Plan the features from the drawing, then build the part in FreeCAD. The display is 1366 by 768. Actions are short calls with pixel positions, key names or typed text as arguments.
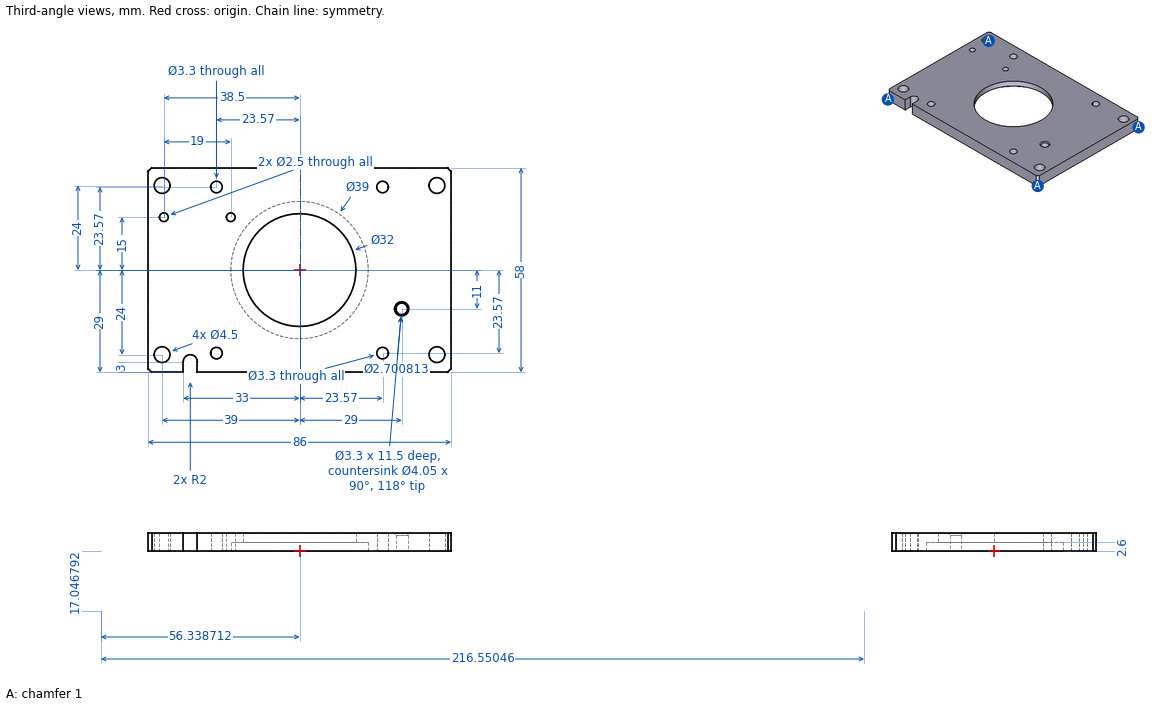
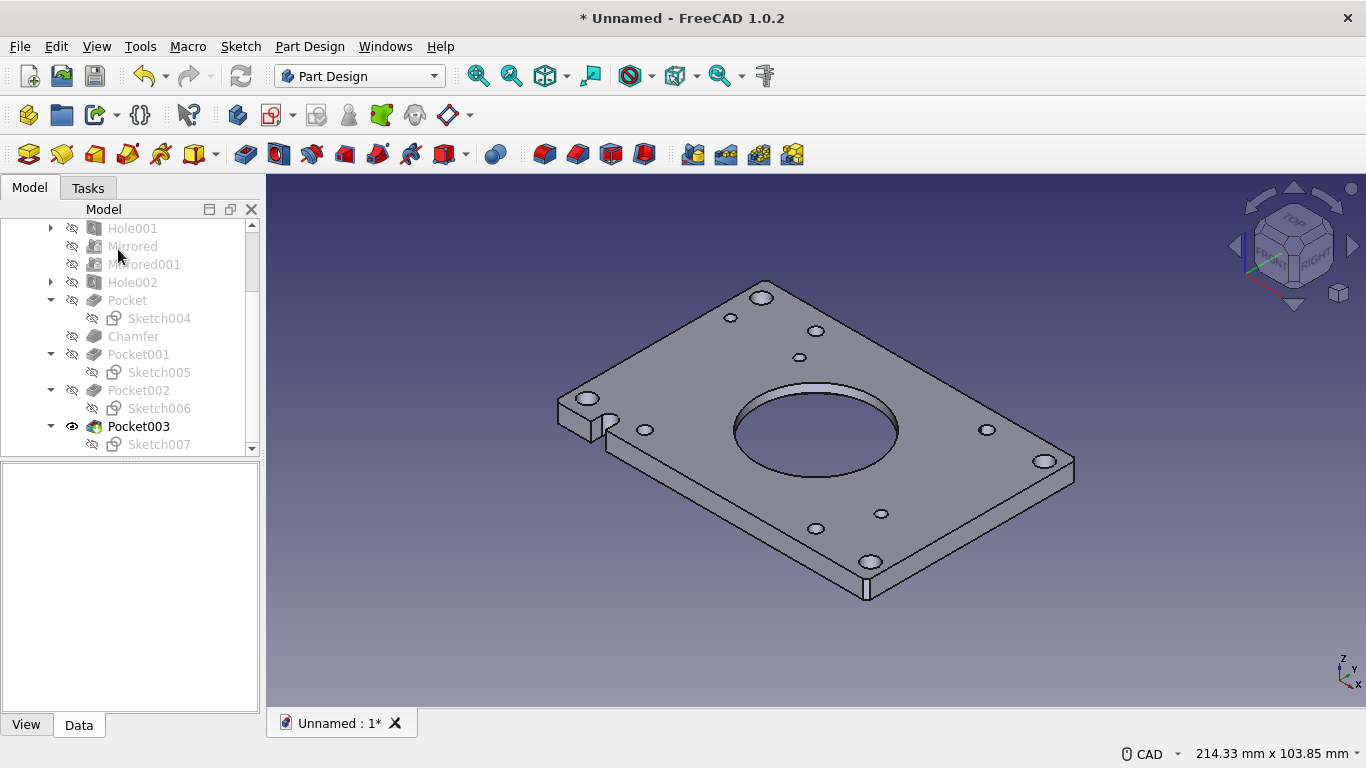
click(697, 395)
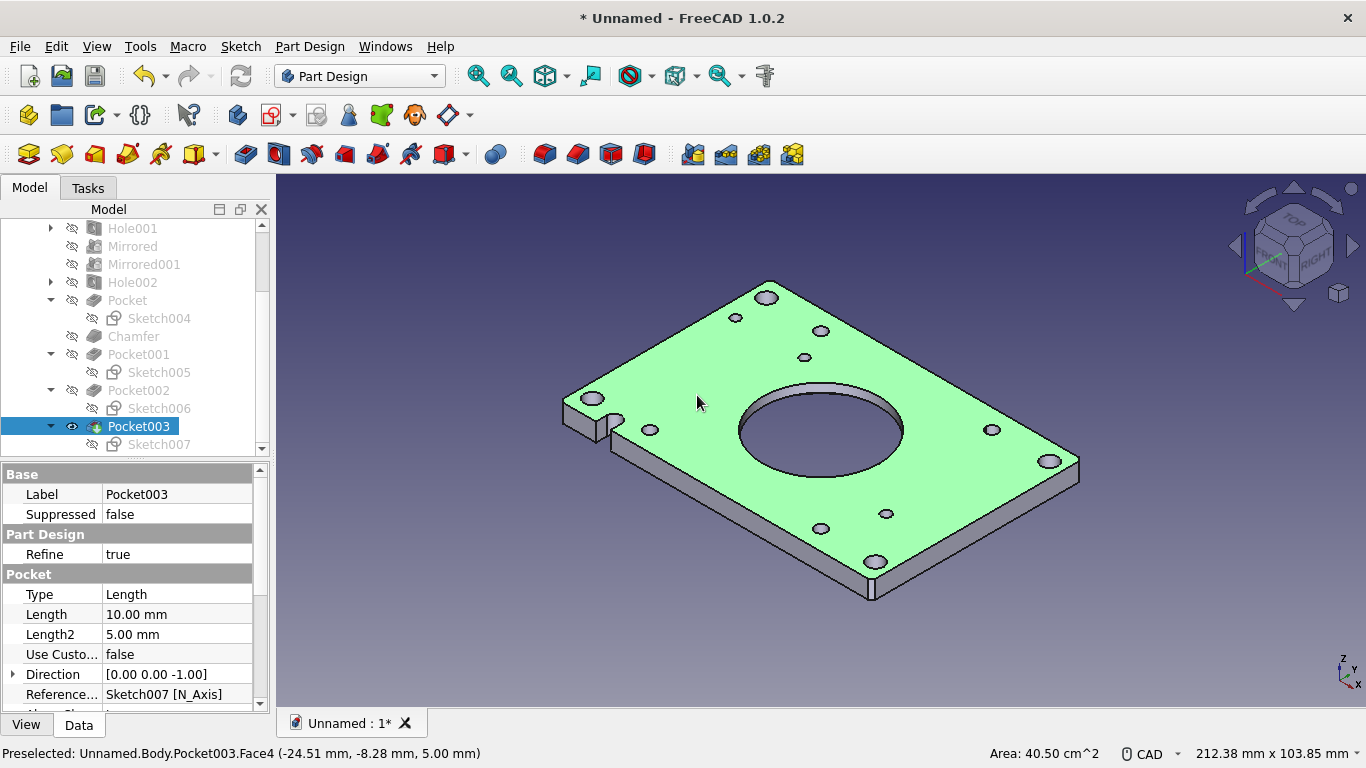
click(270, 116)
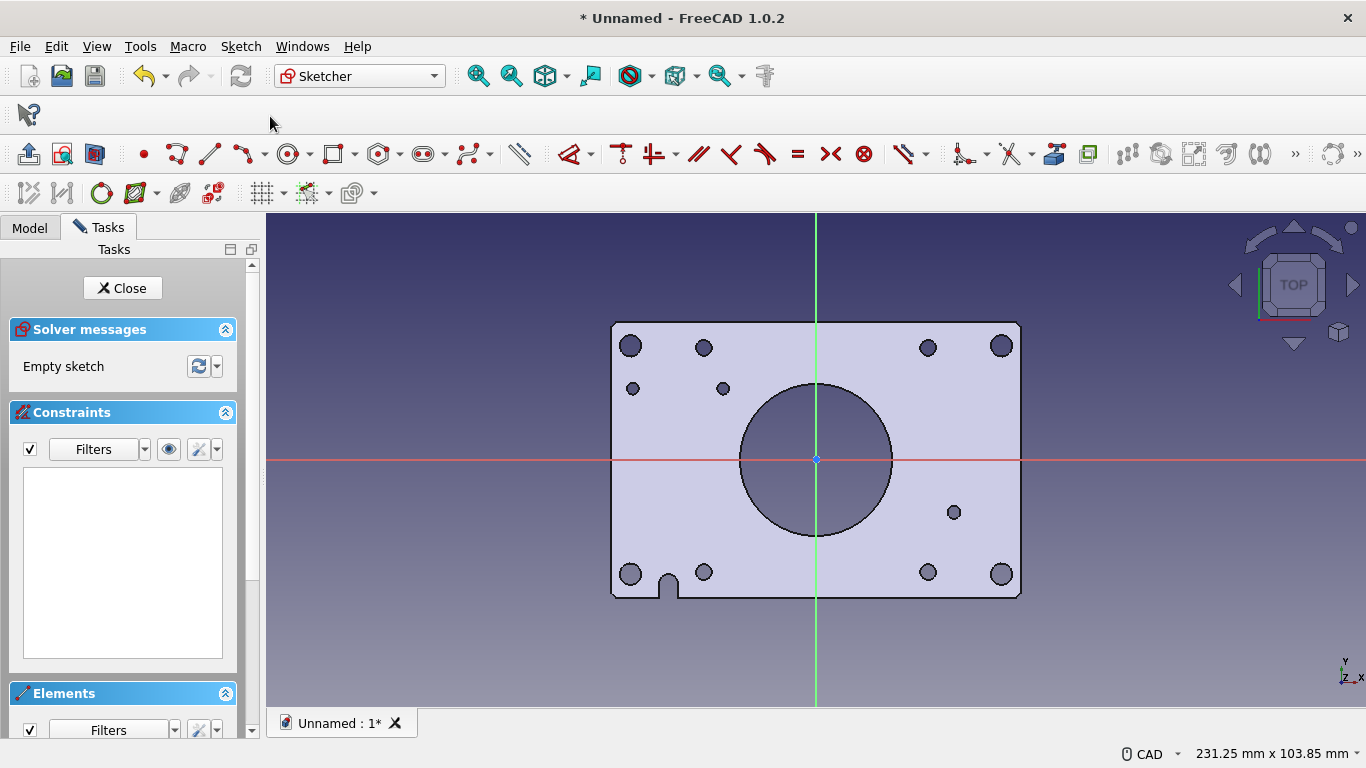
scroll(965, 515, up, 15)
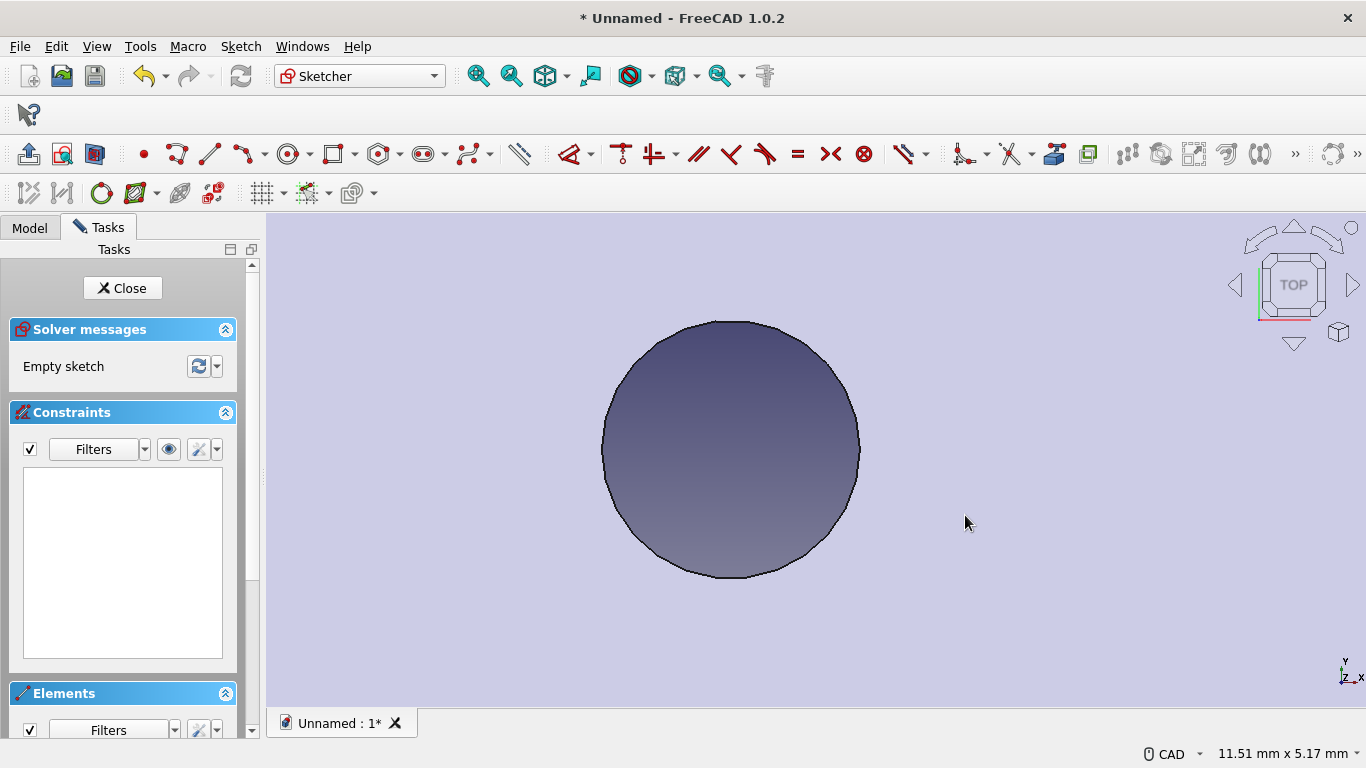
key(g)
key(c)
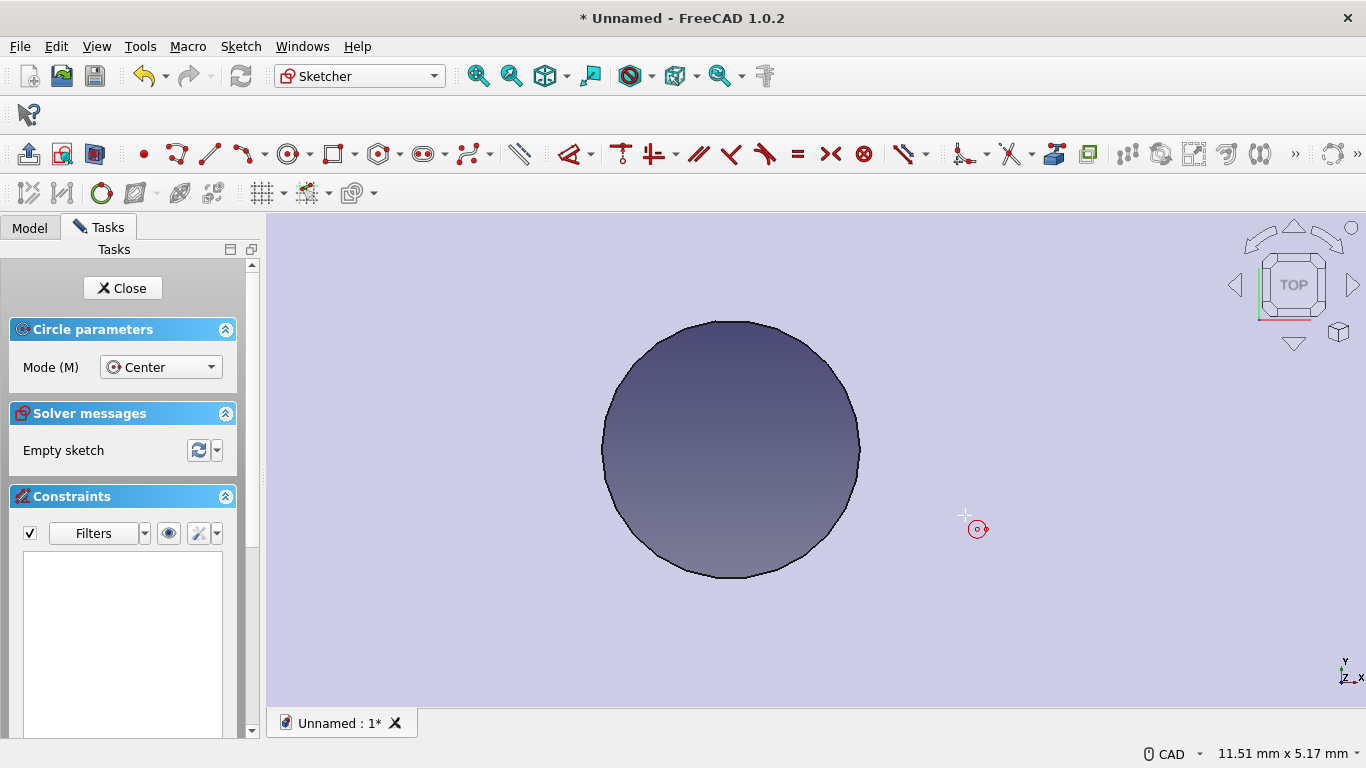
click(731, 450)
move(842, 338)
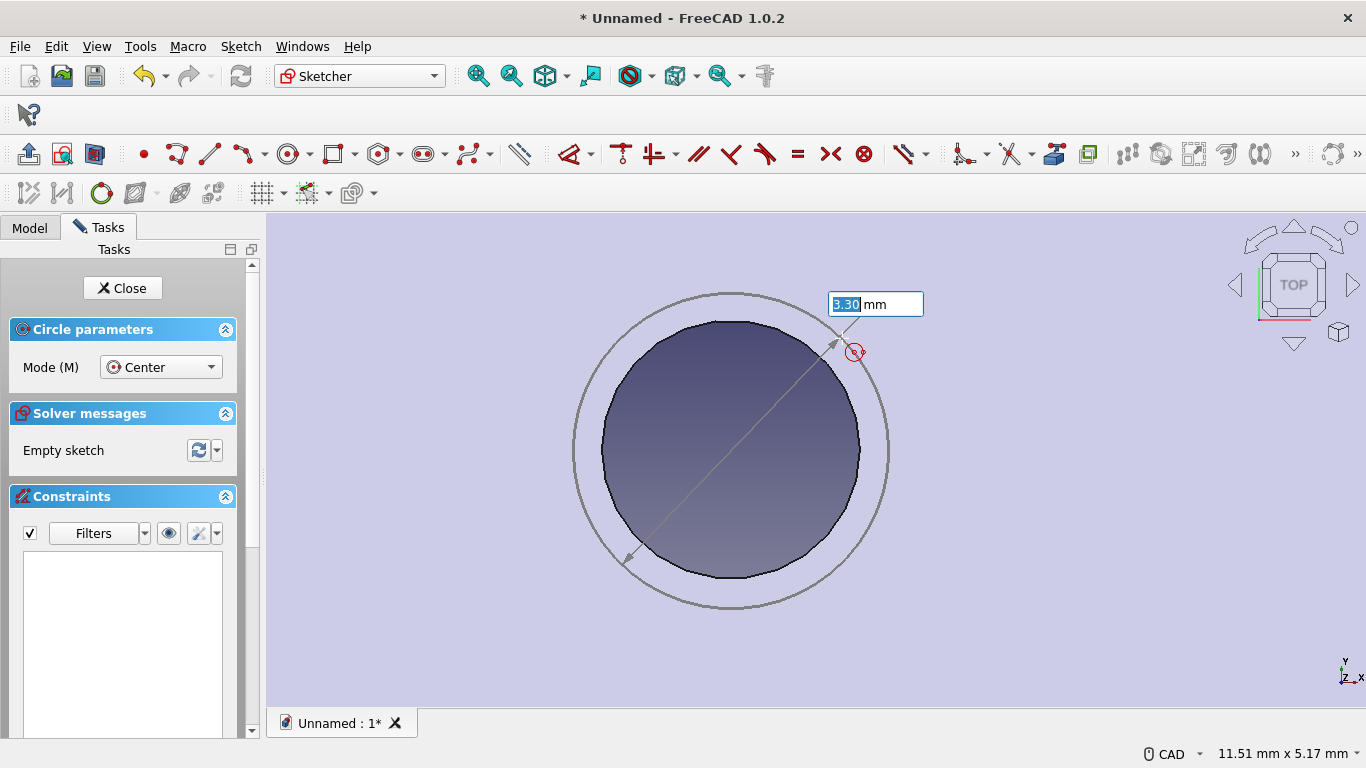
text(3.3)
key(Return)
key(Escape)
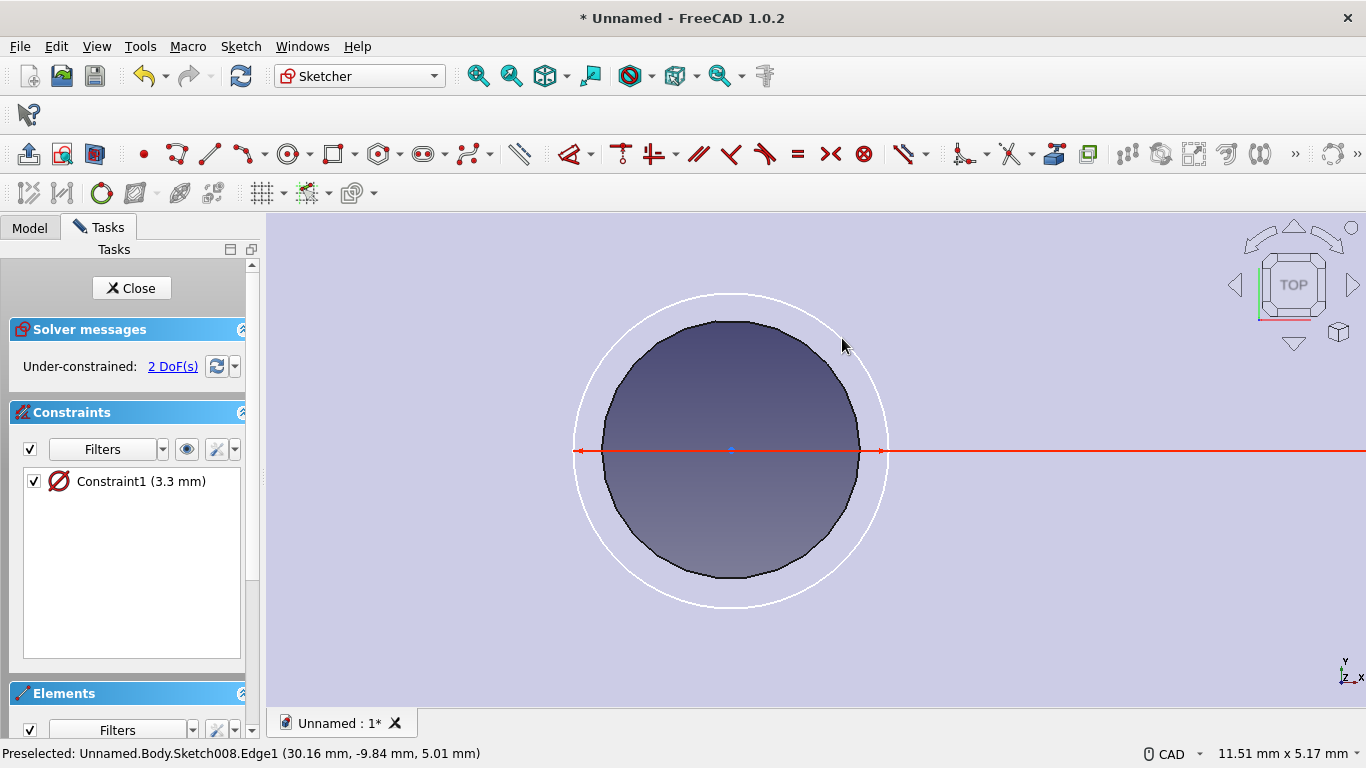
key(d)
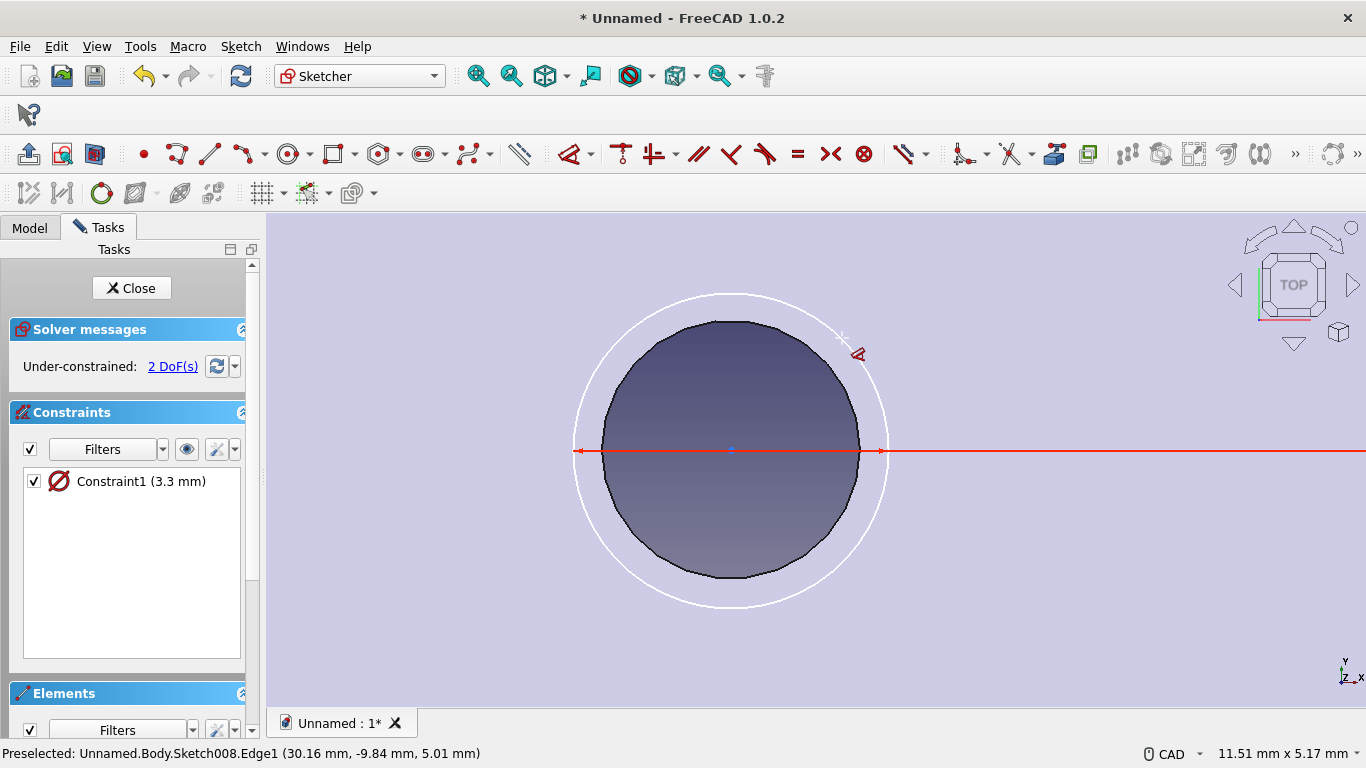
click(731, 451)
click(513, 485)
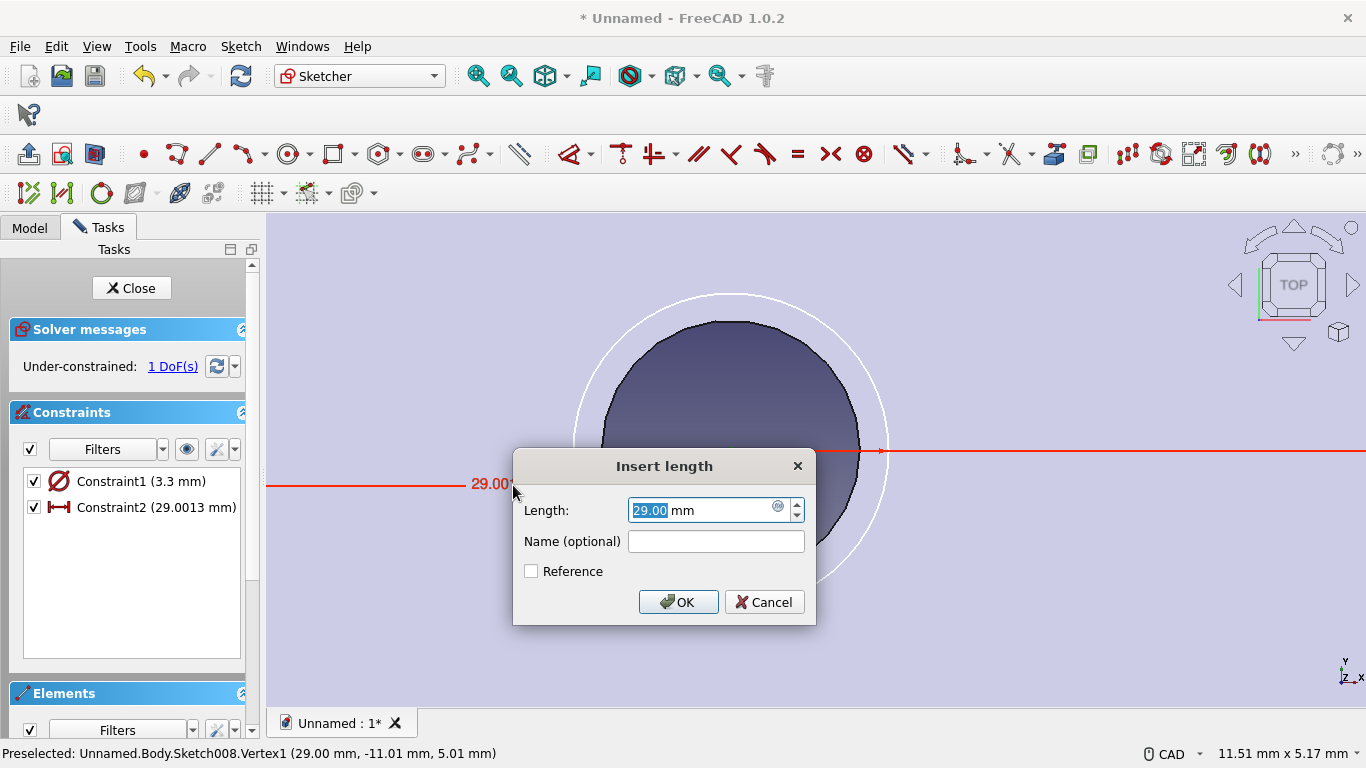
text(29)
key(Return)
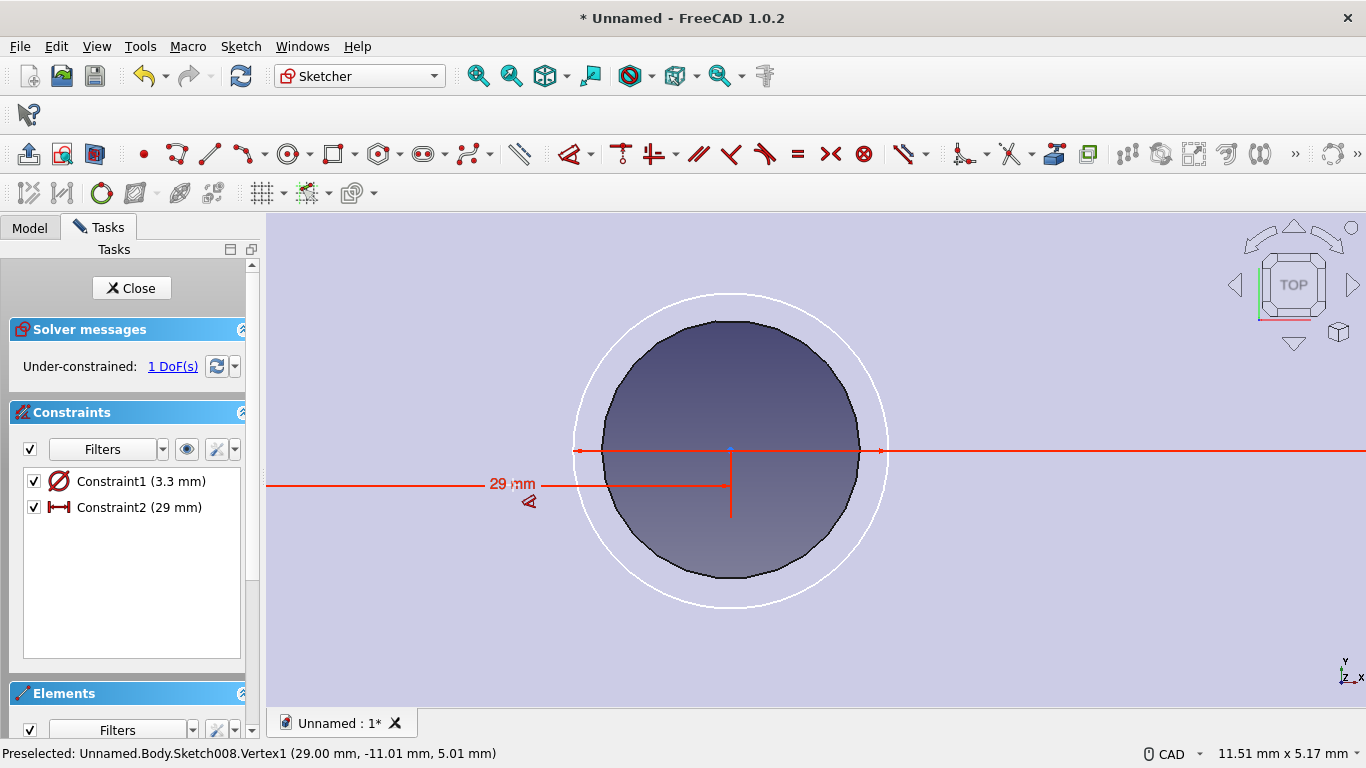
click(731, 451)
click(765, 346)